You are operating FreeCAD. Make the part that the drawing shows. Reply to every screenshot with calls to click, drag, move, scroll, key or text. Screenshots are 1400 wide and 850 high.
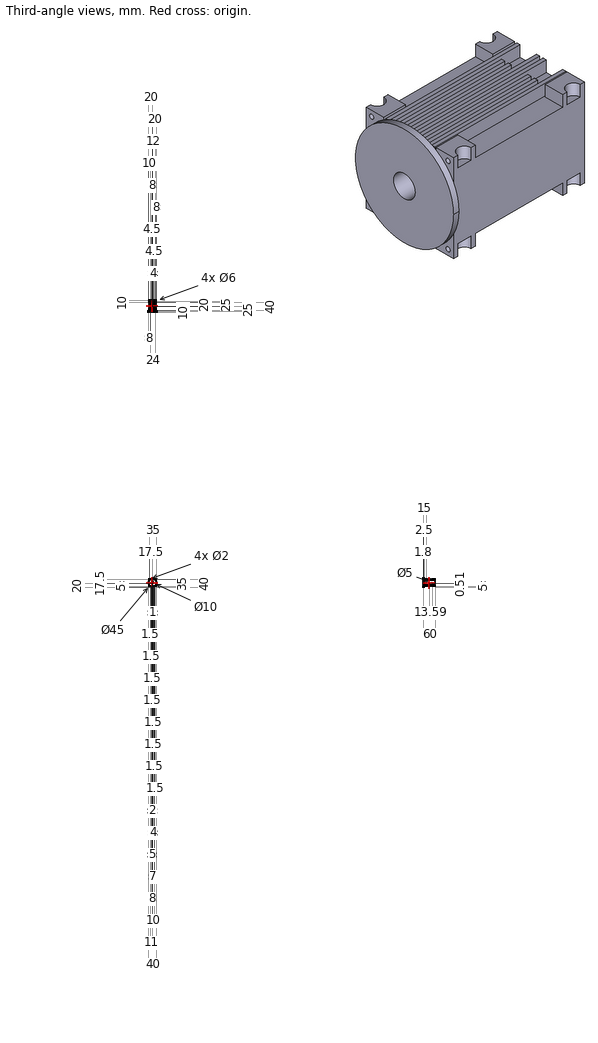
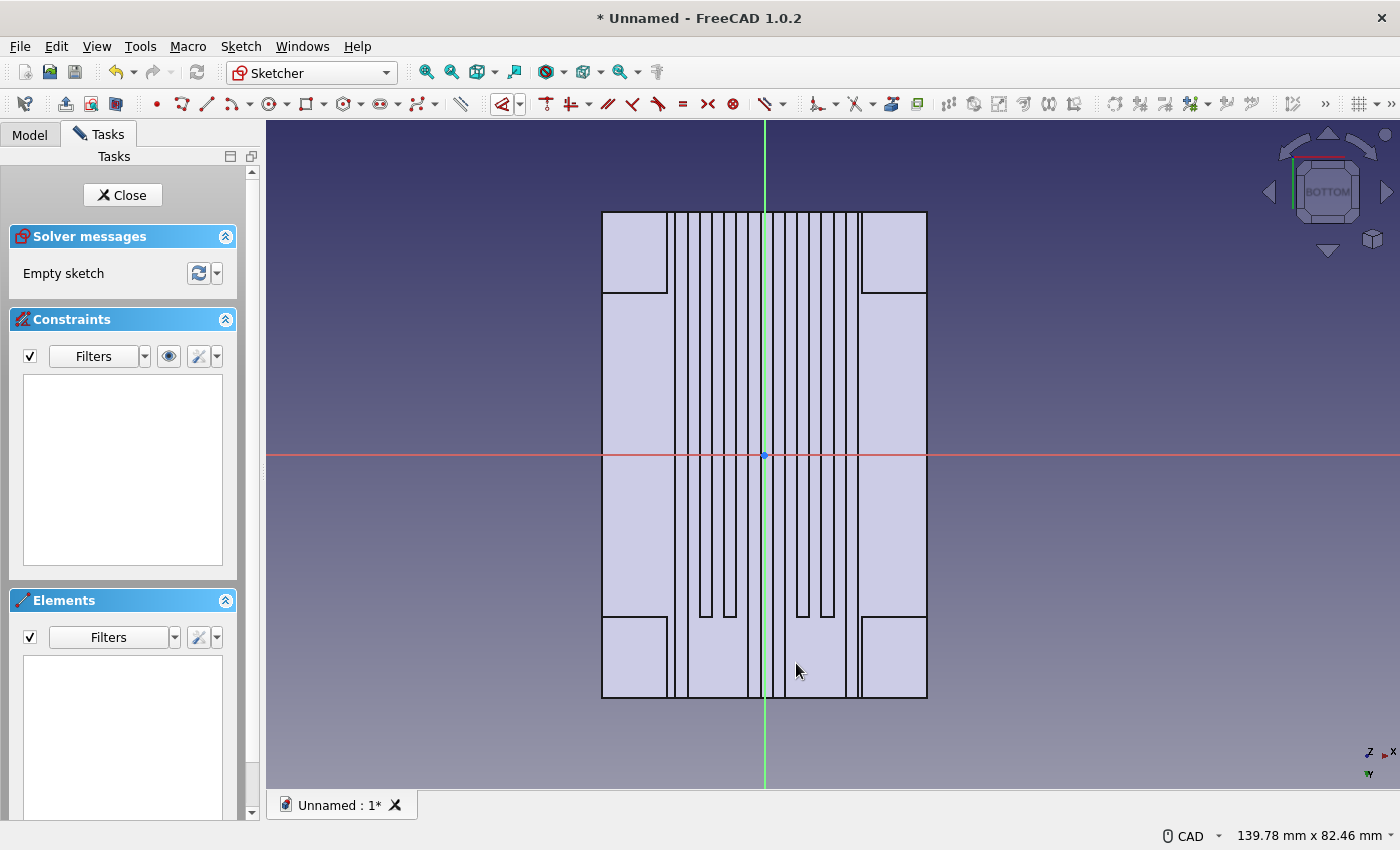
key(g)
key(c)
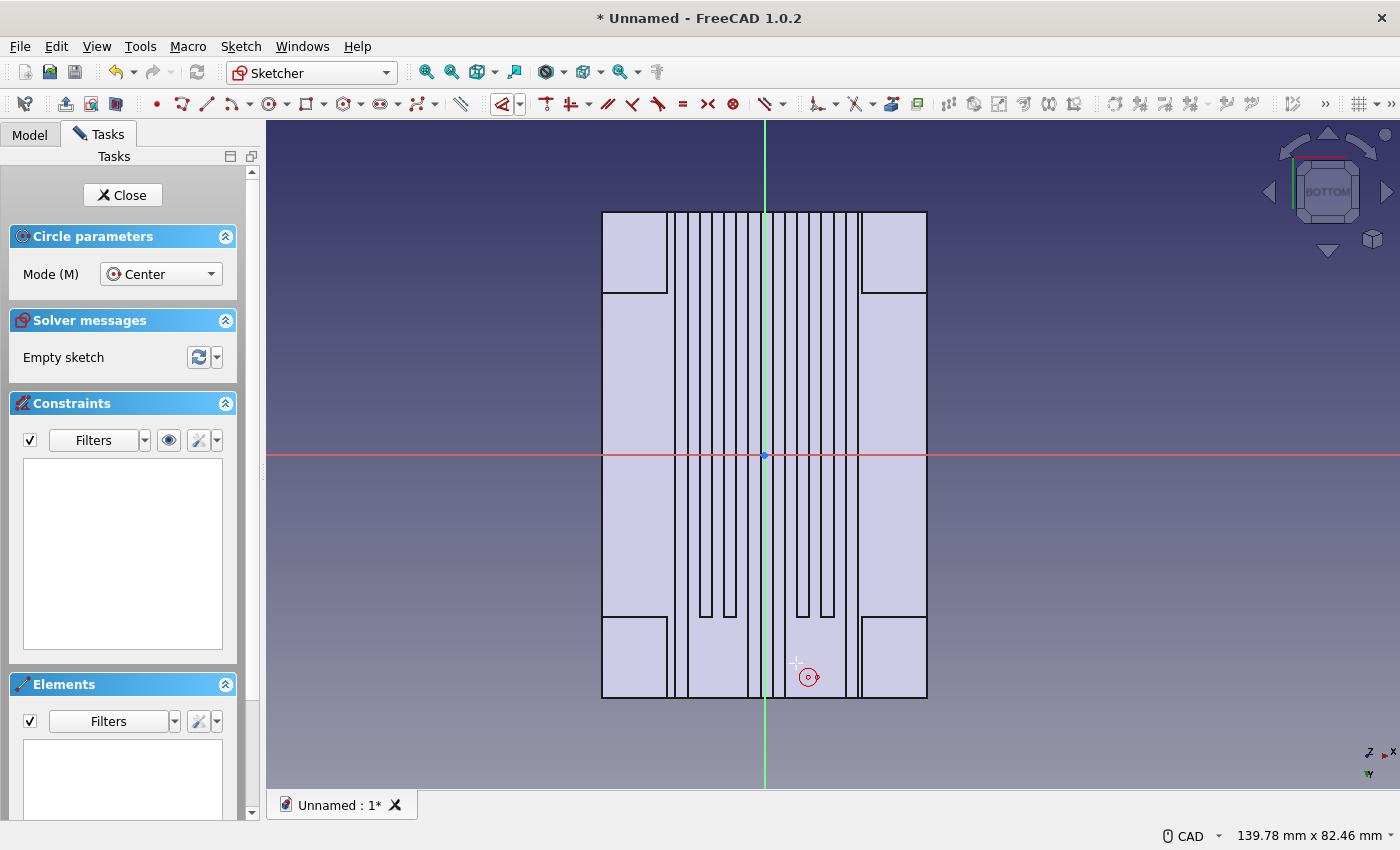
click(927, 658)
click(944, 641)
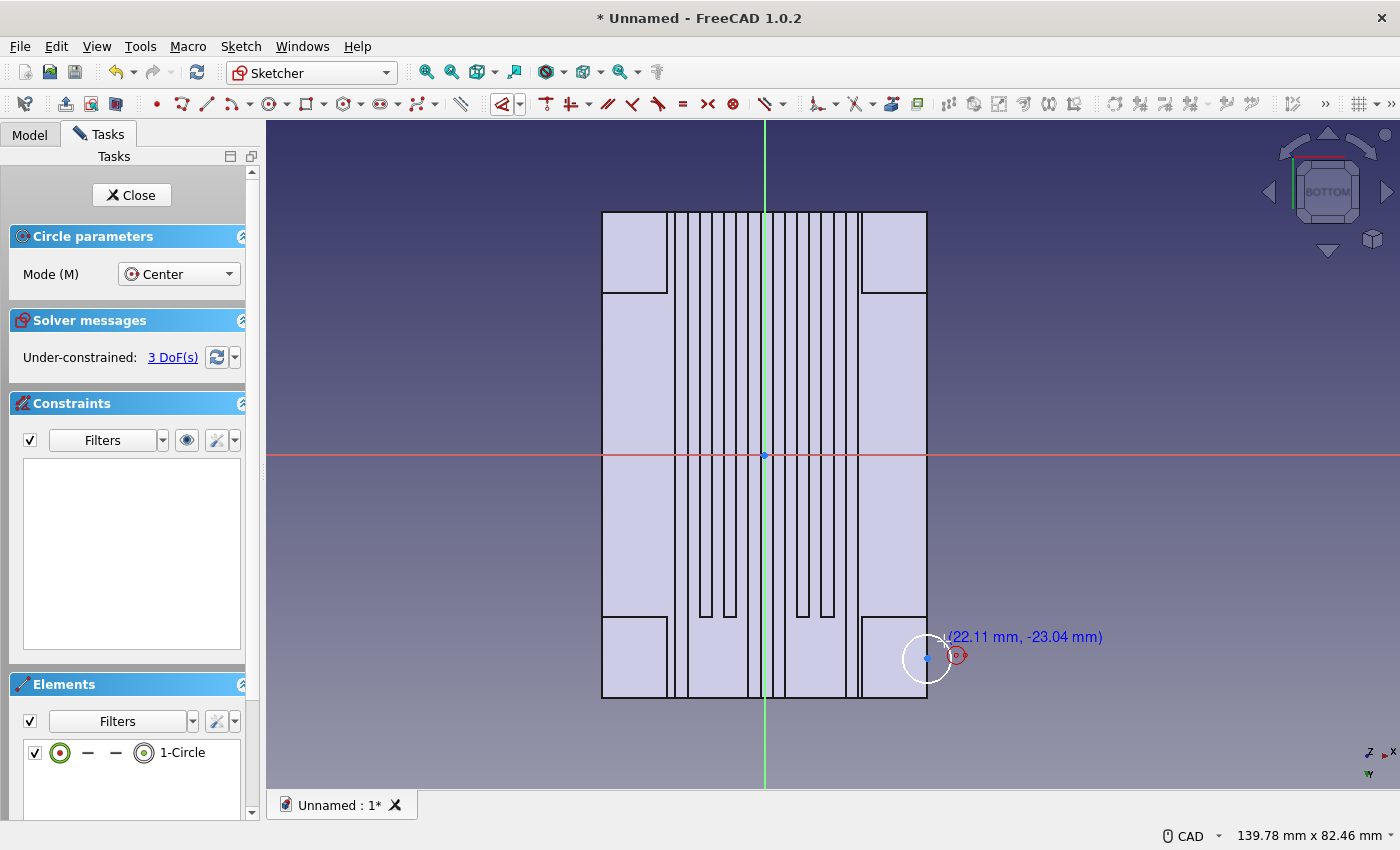
click(602, 658)
click(620, 641)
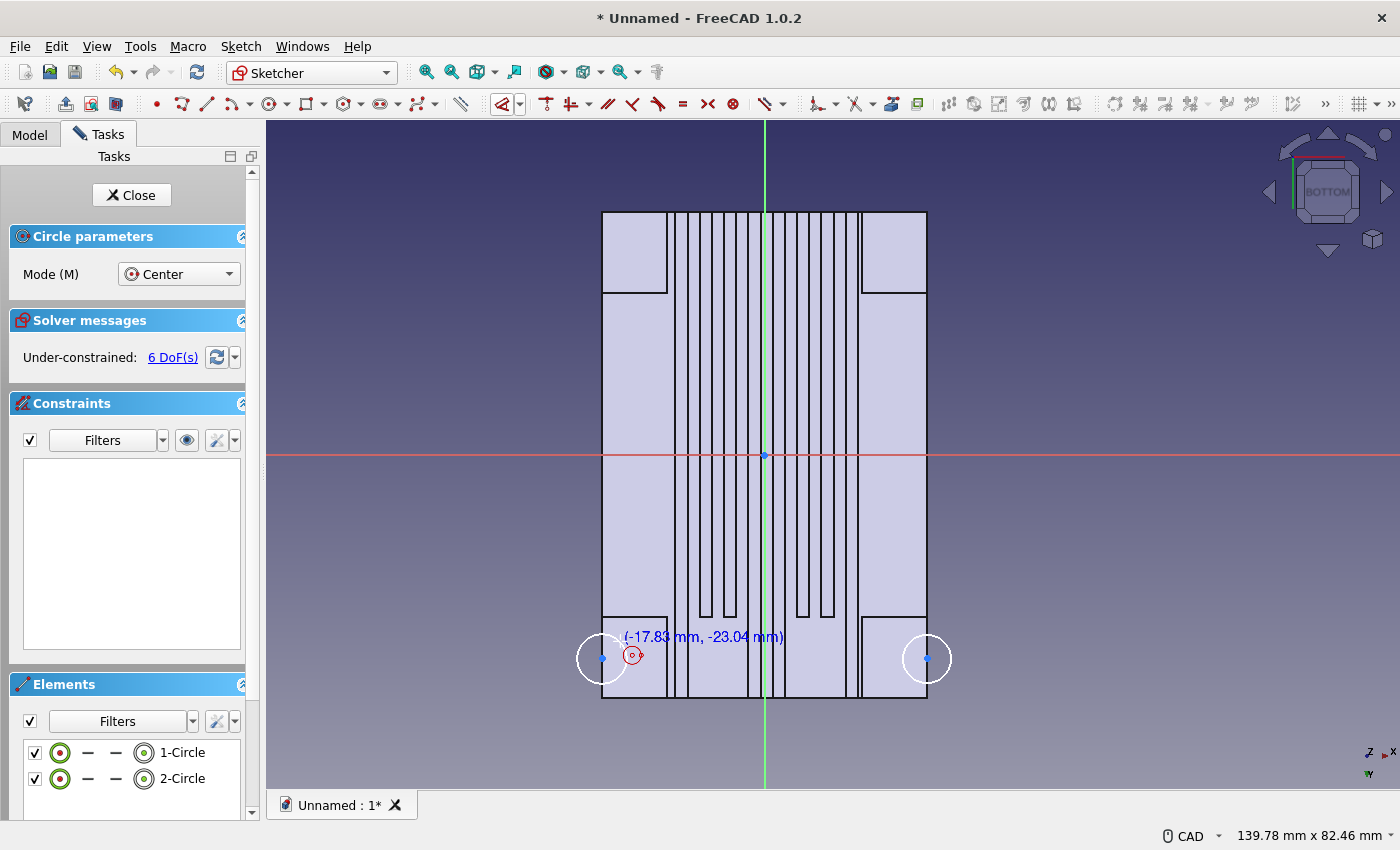
click(927, 252)
click(944, 235)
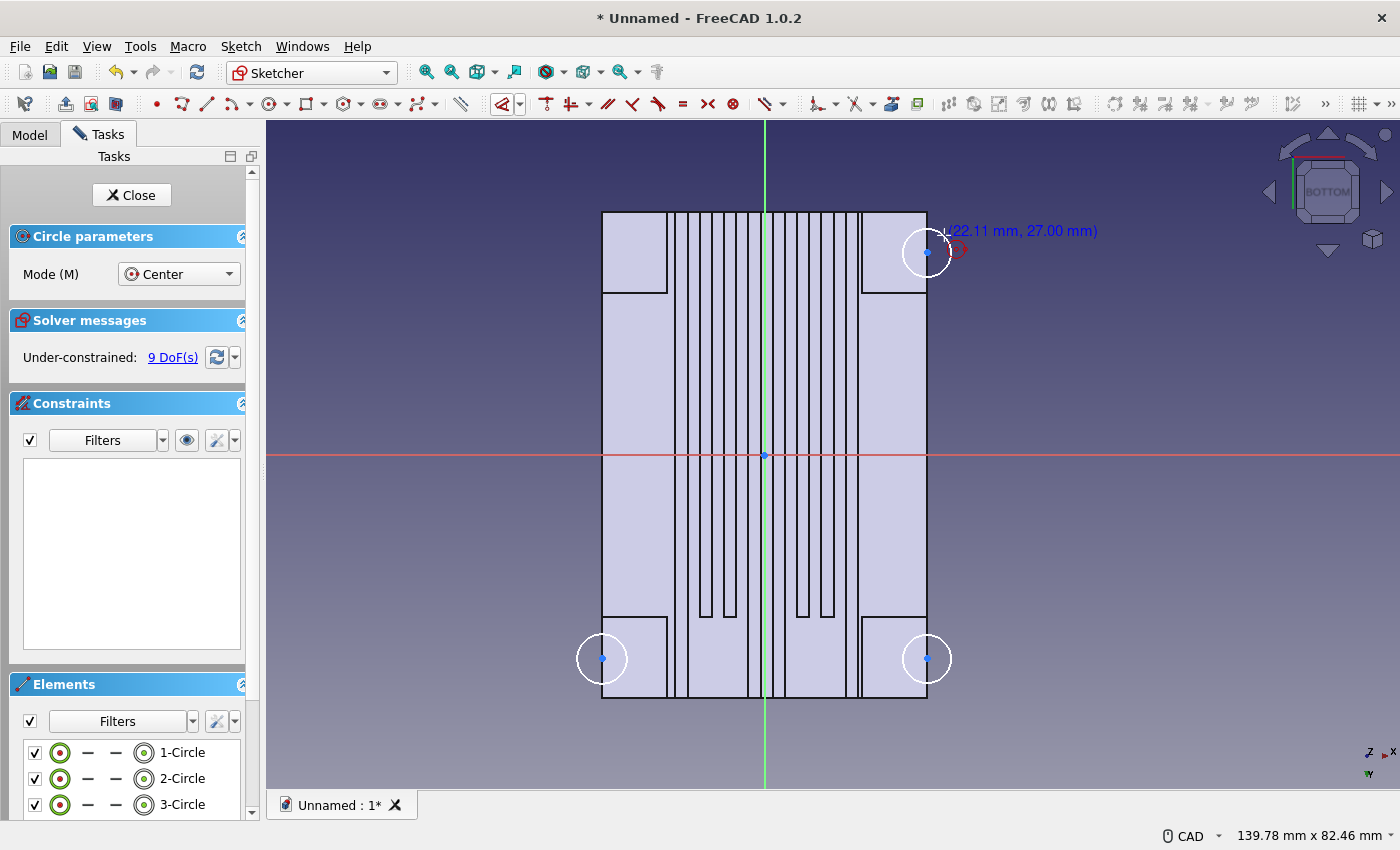
click(602, 252)
click(620, 235)
key(Escape)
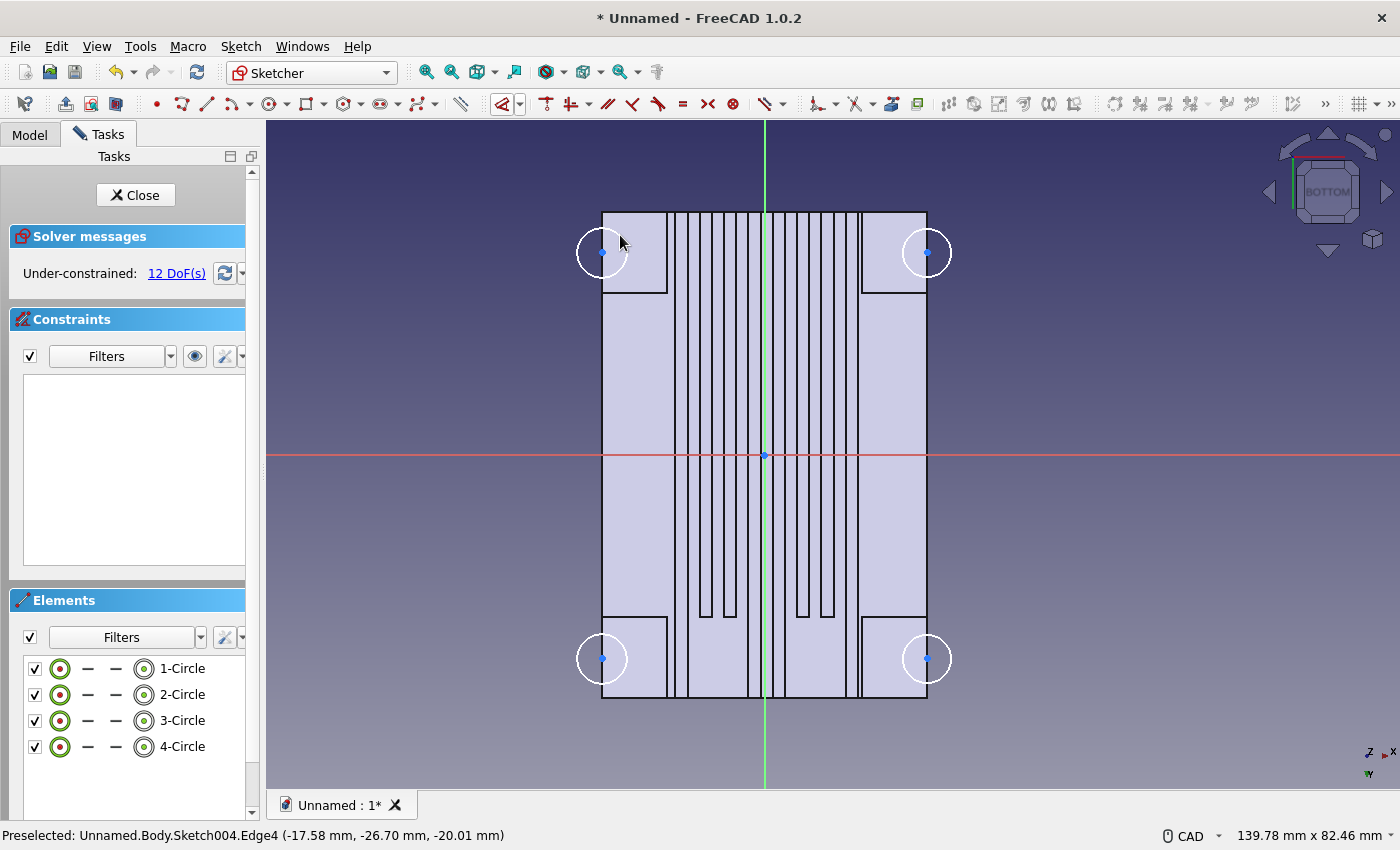
click(944, 642)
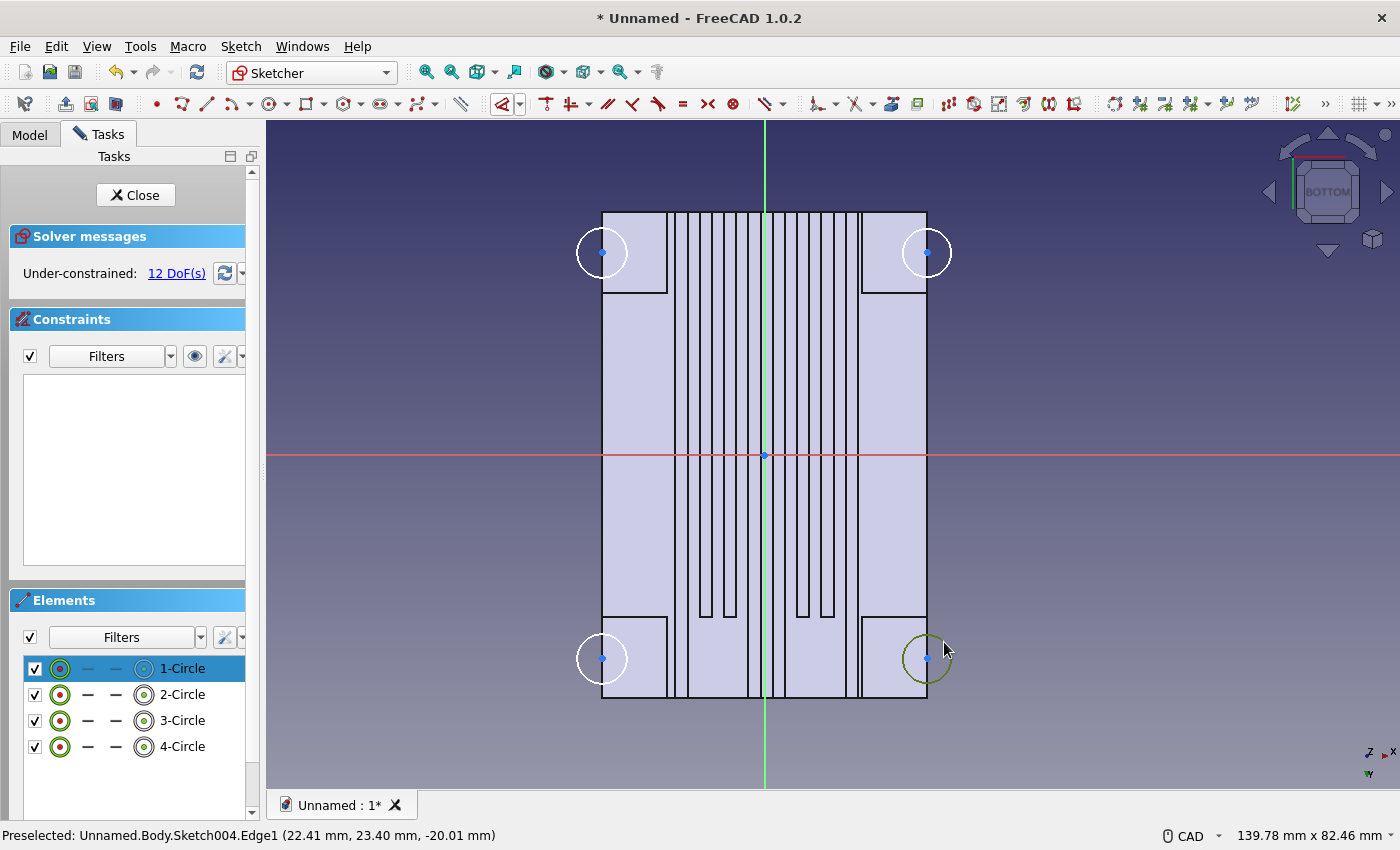
click(619, 641)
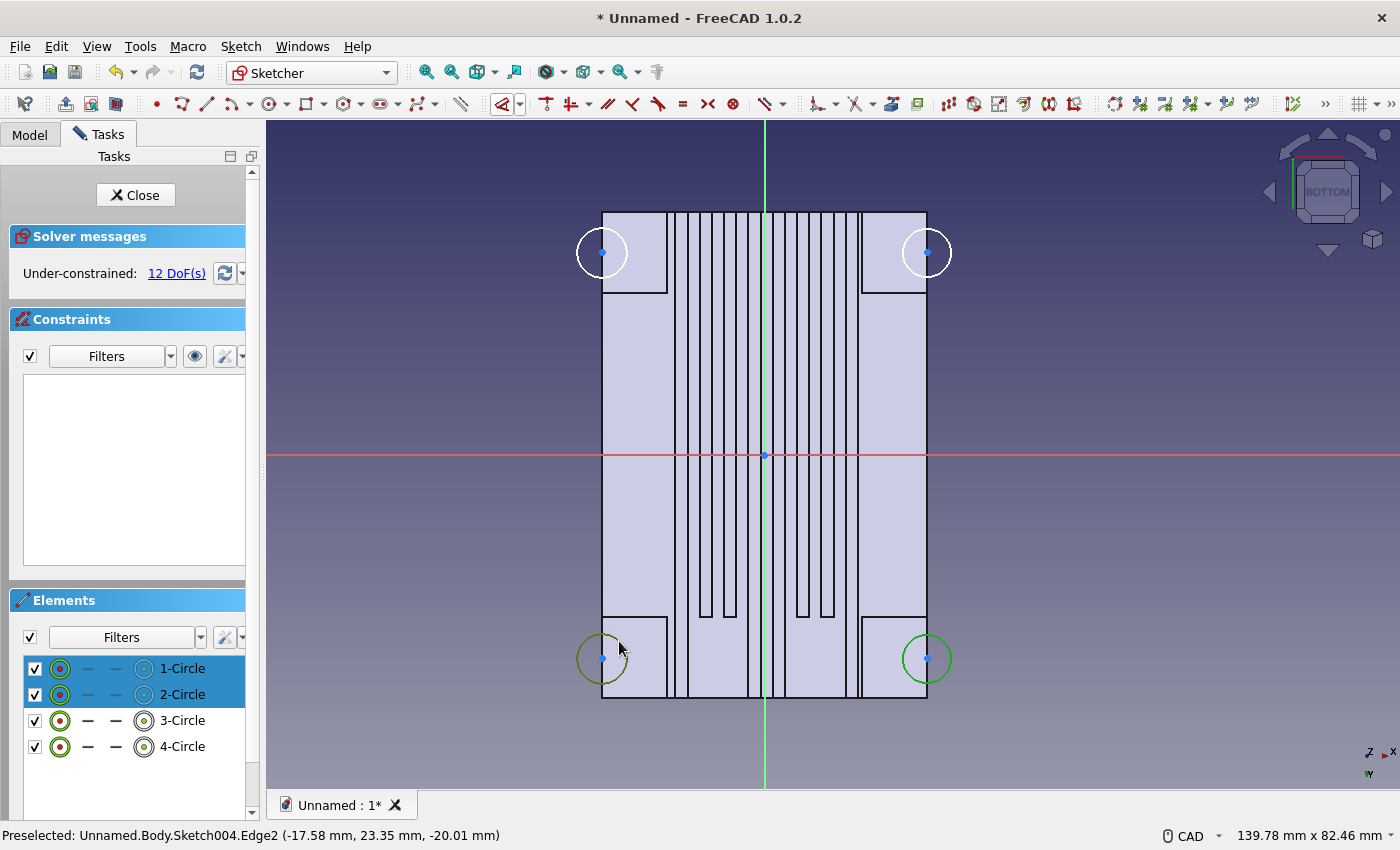
click(944, 236)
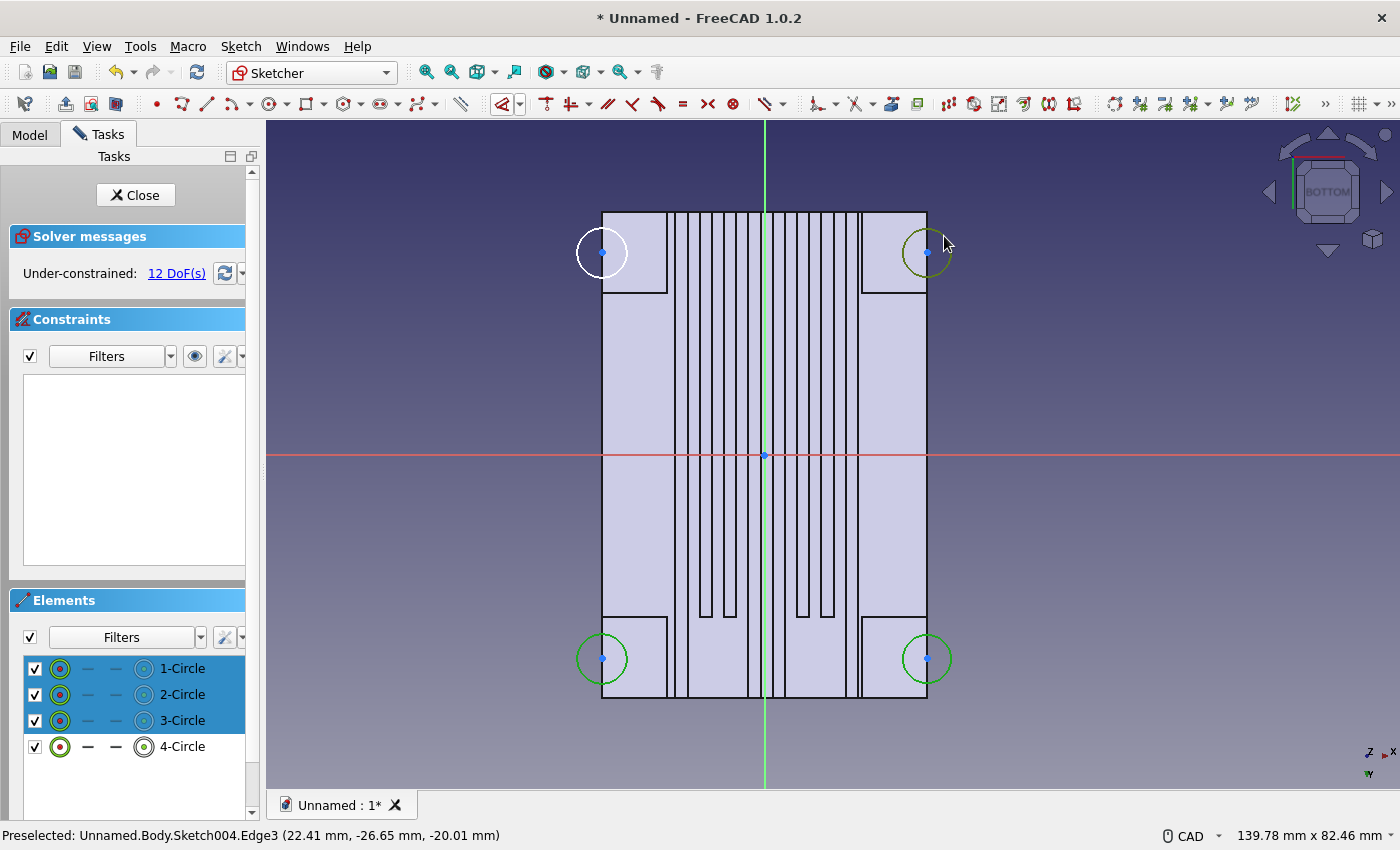
click(619, 235)